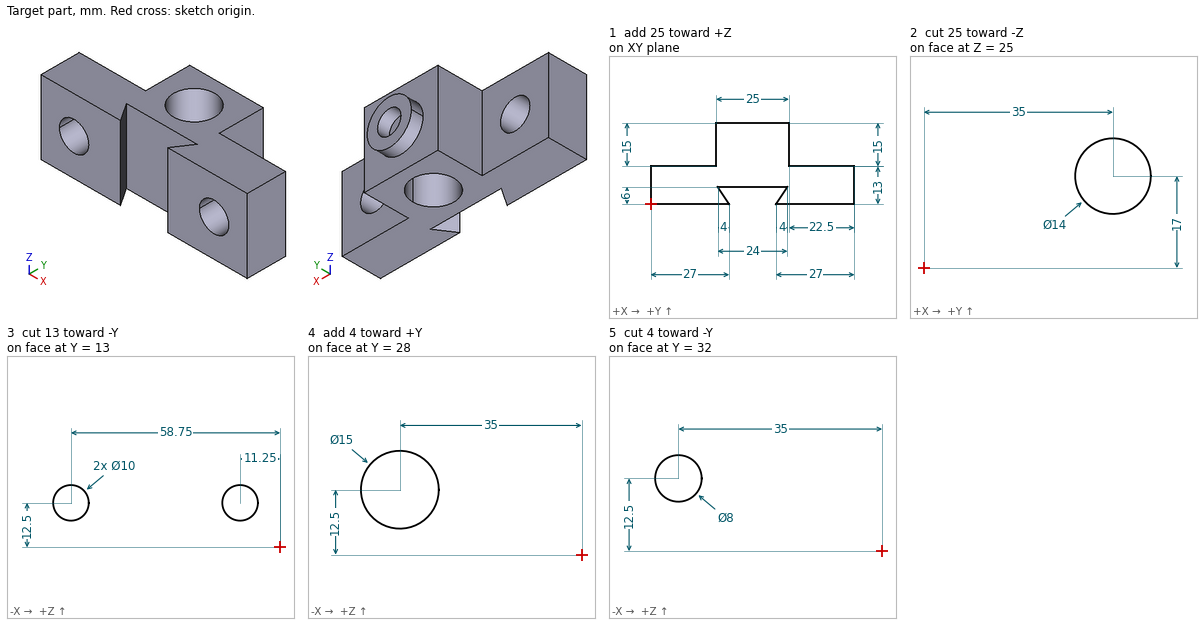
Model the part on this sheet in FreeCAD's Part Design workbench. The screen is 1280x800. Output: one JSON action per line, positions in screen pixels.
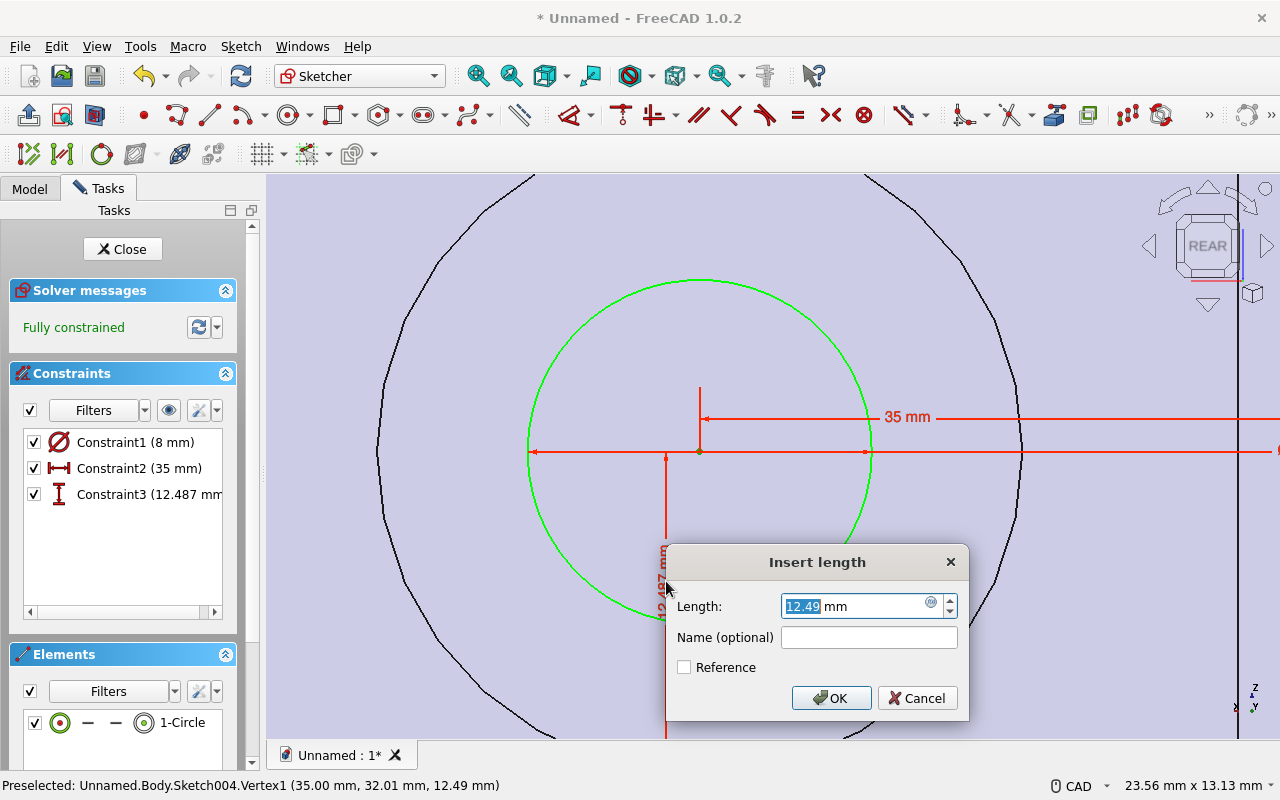
{"action": "type", "text": "12.5"}
{"action": "key", "text": "Return"}
{"action": "key", "text": "Escape"}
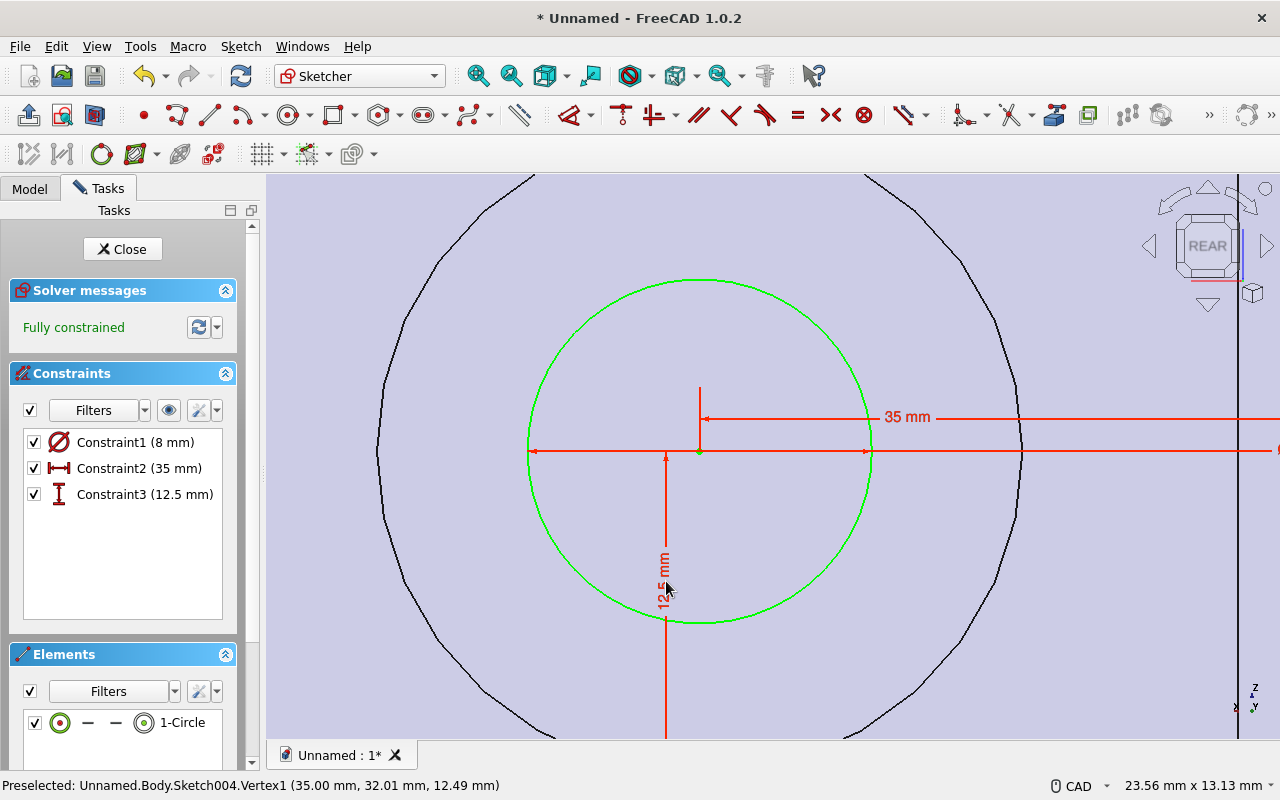
{"action": "left_click", "coordinate": [123, 249]}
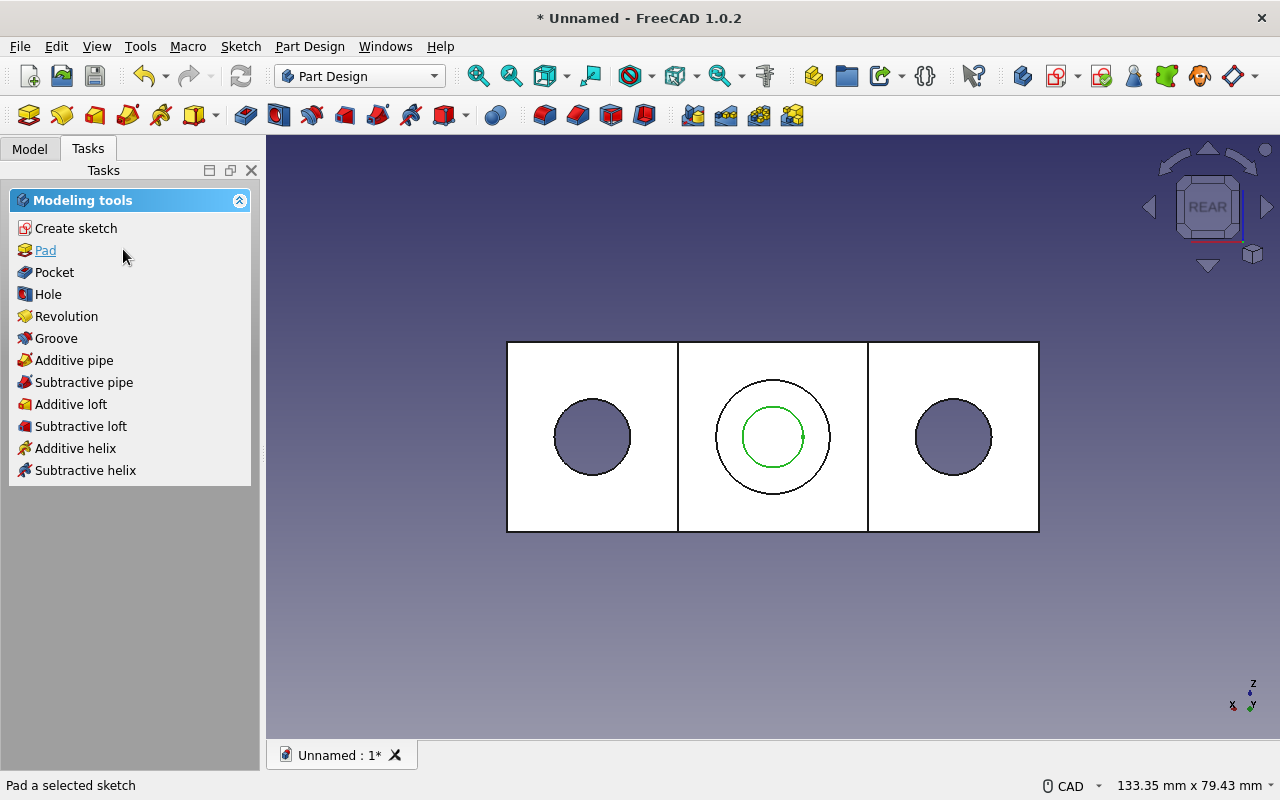
{"action": "left_click", "coordinate": [246, 116]}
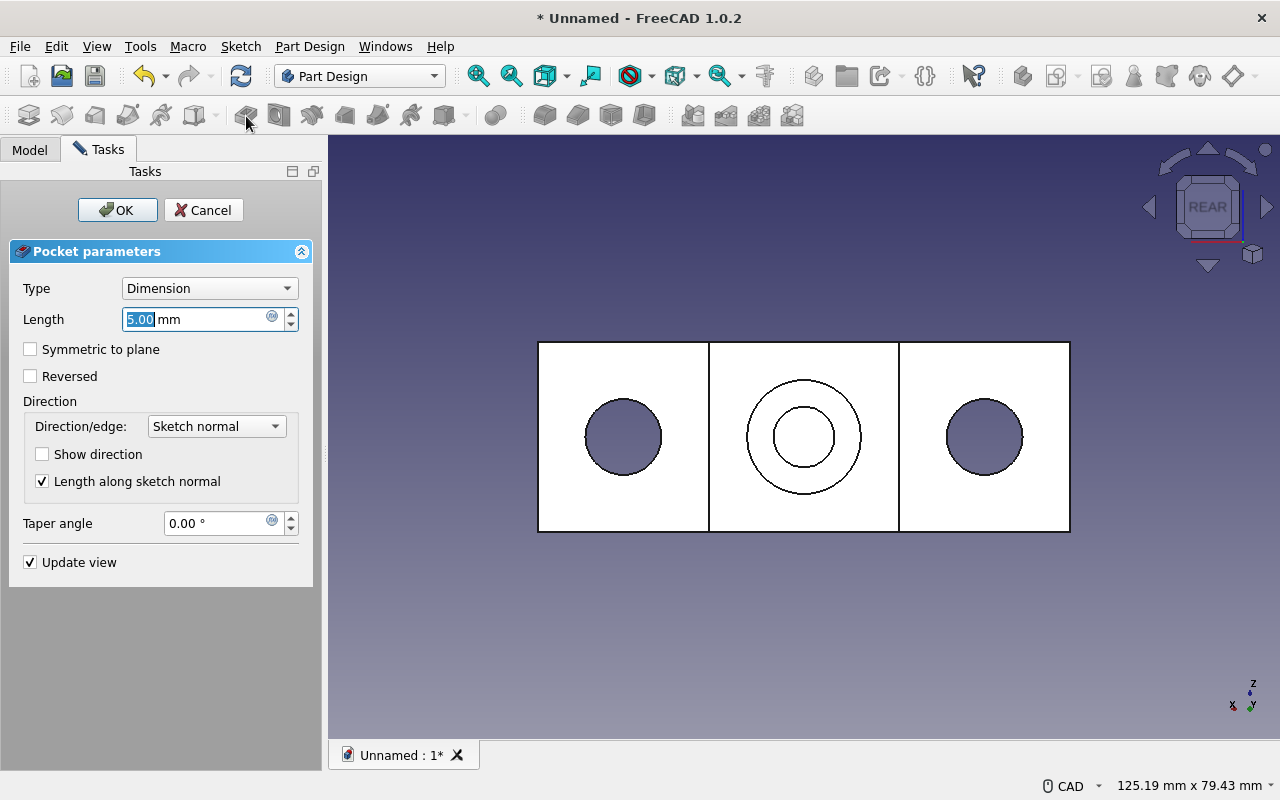
{"action": "type", "text": "4"}
{"action": "key", "text": "Tab"}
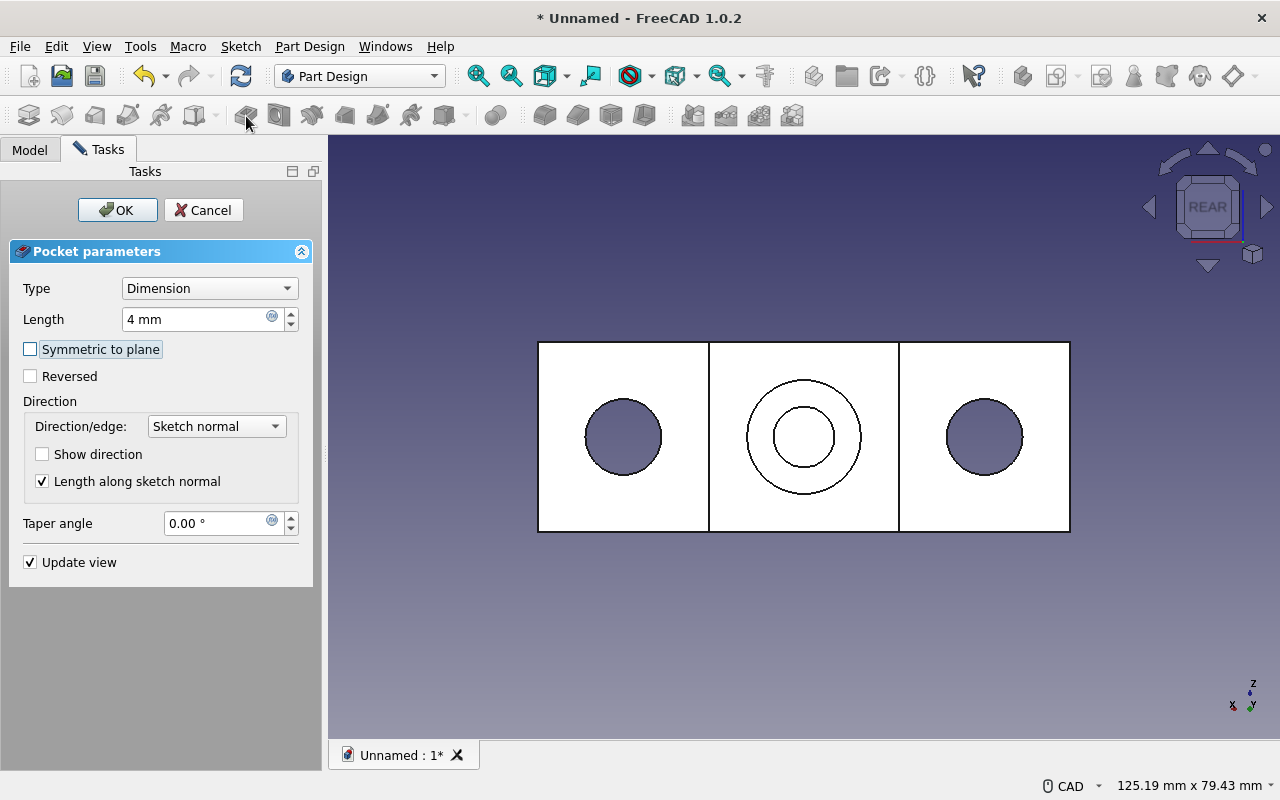
{"action": "left_click", "coordinate": [118, 210]}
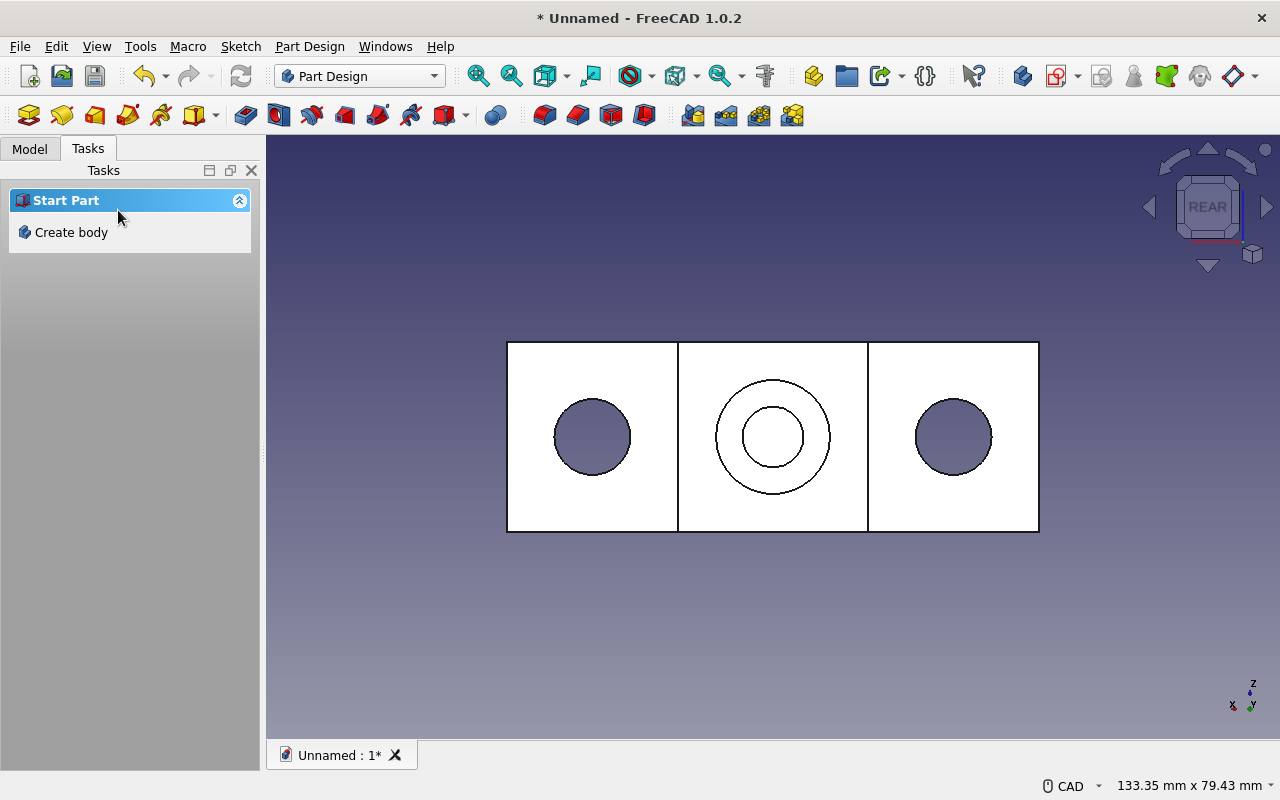
{"action": "key", "text": "0"}